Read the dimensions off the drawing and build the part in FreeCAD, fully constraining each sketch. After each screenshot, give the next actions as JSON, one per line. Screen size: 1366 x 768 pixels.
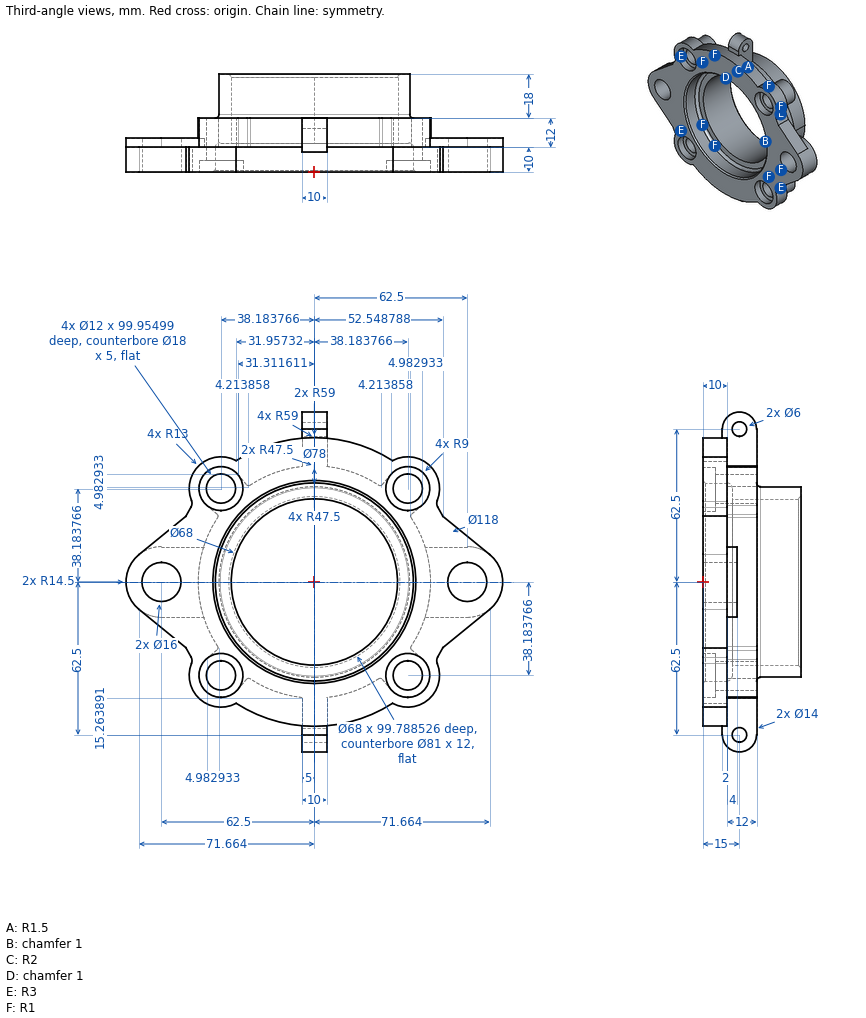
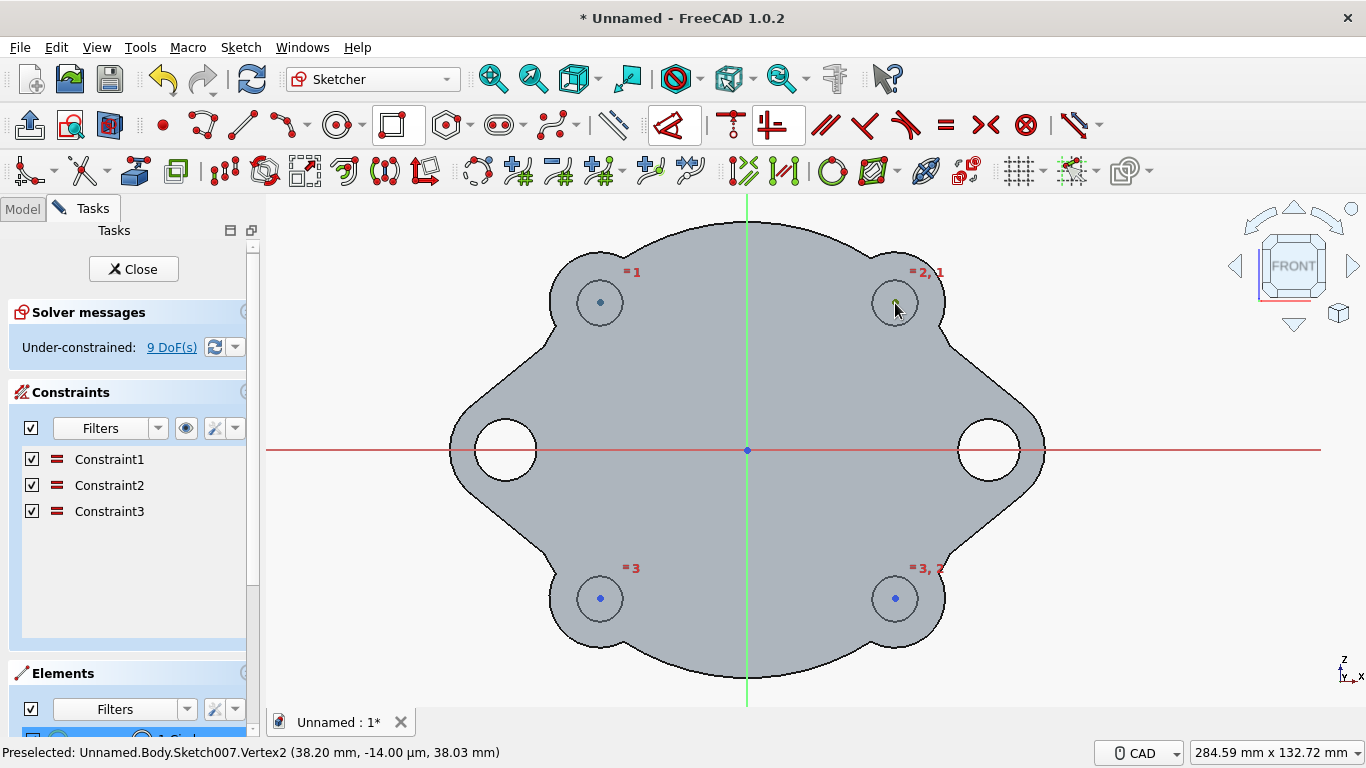
{"action": "key", "text": "h"}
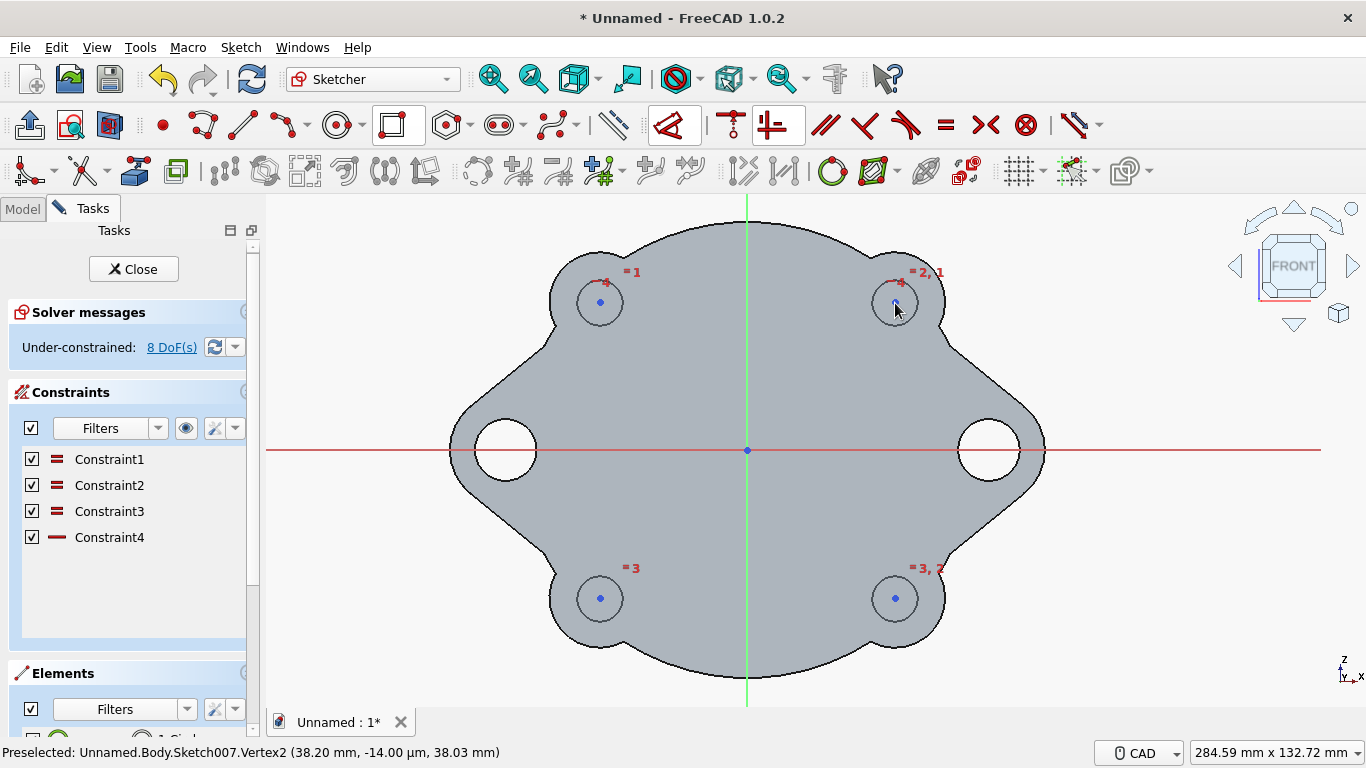
{"action": "left_click", "coordinate": [895, 303]}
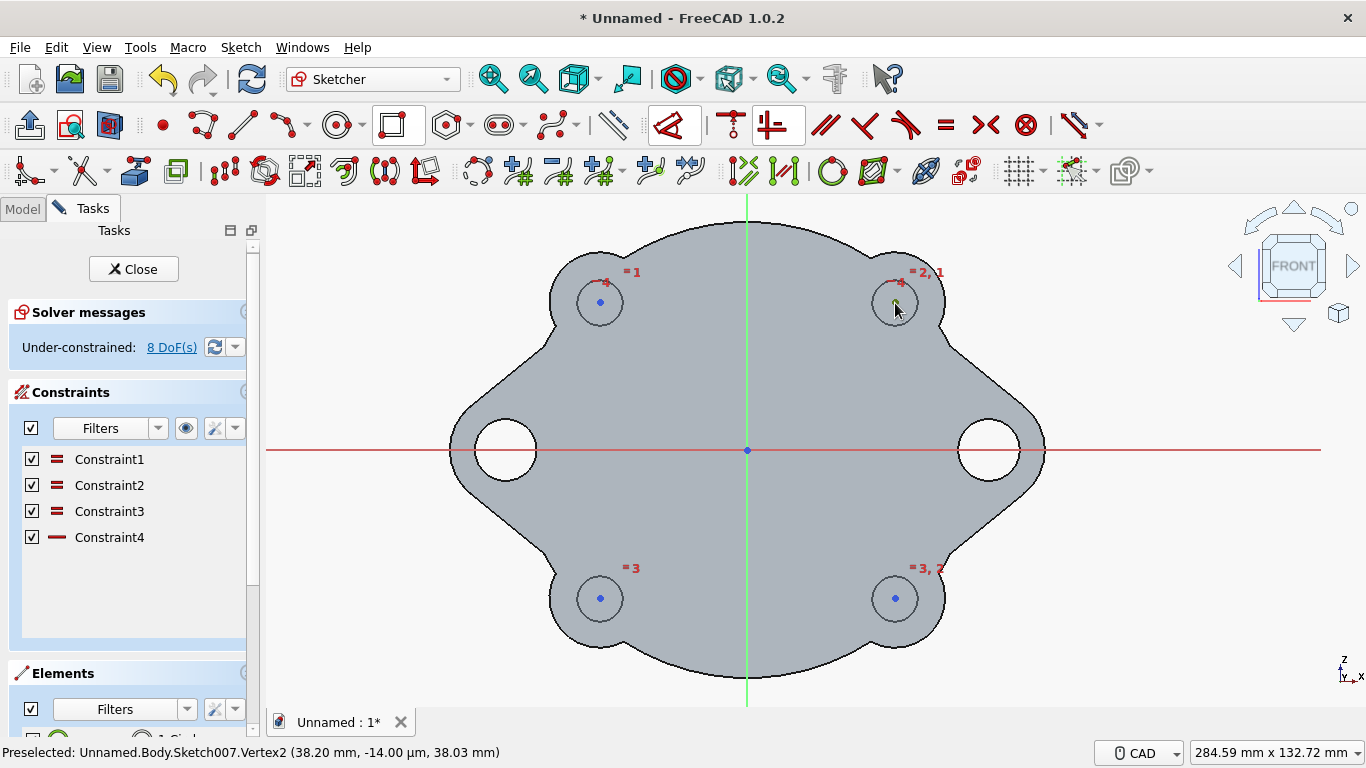
{"action": "left_click", "coordinate": [895, 599]}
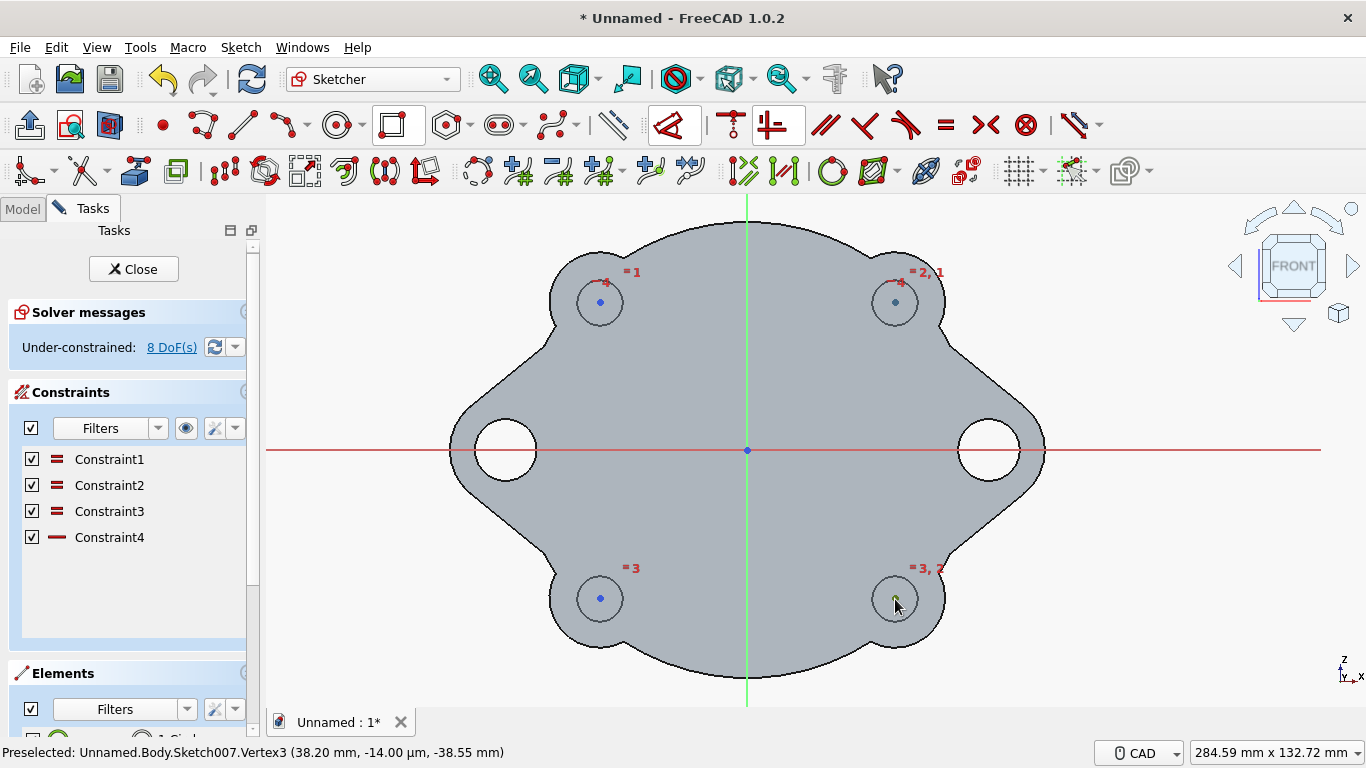
{"action": "key", "text": "v"}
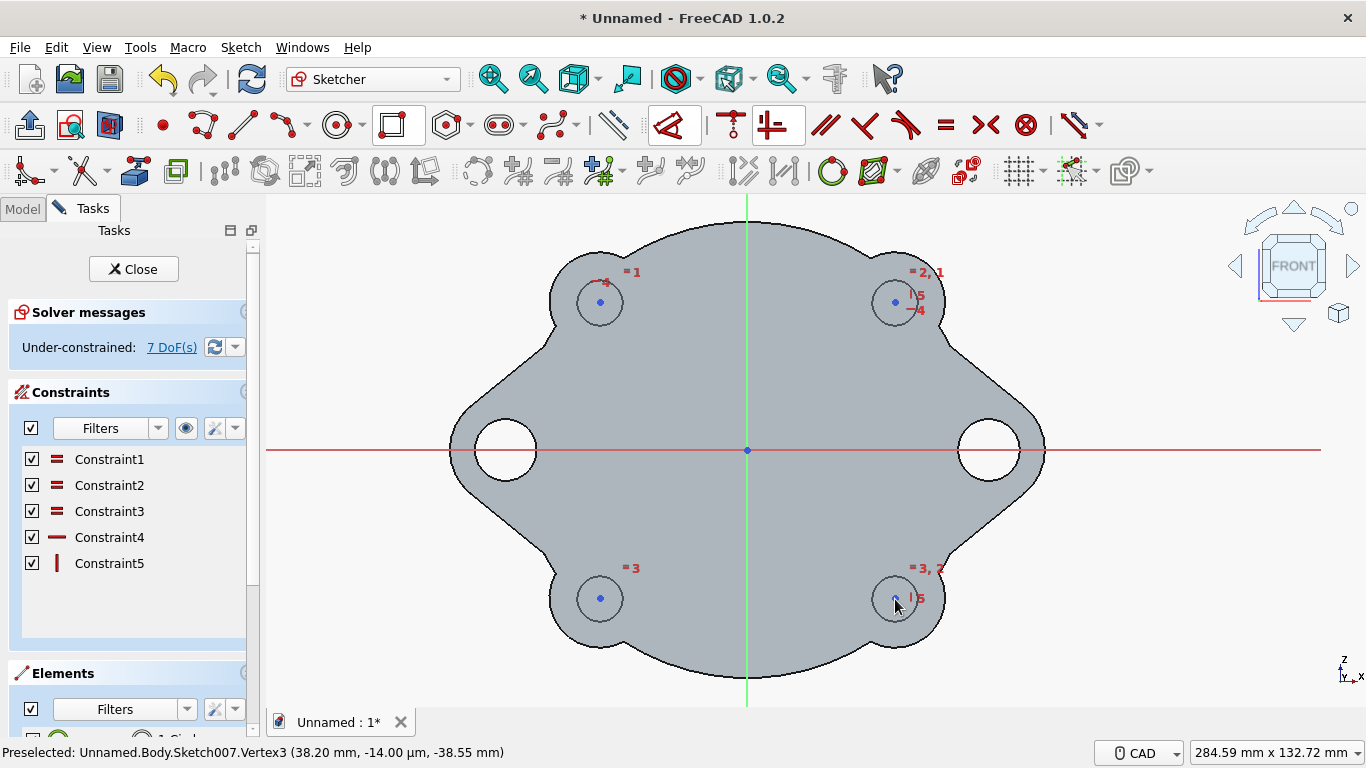
{"action": "left_click", "coordinate": [600, 303]}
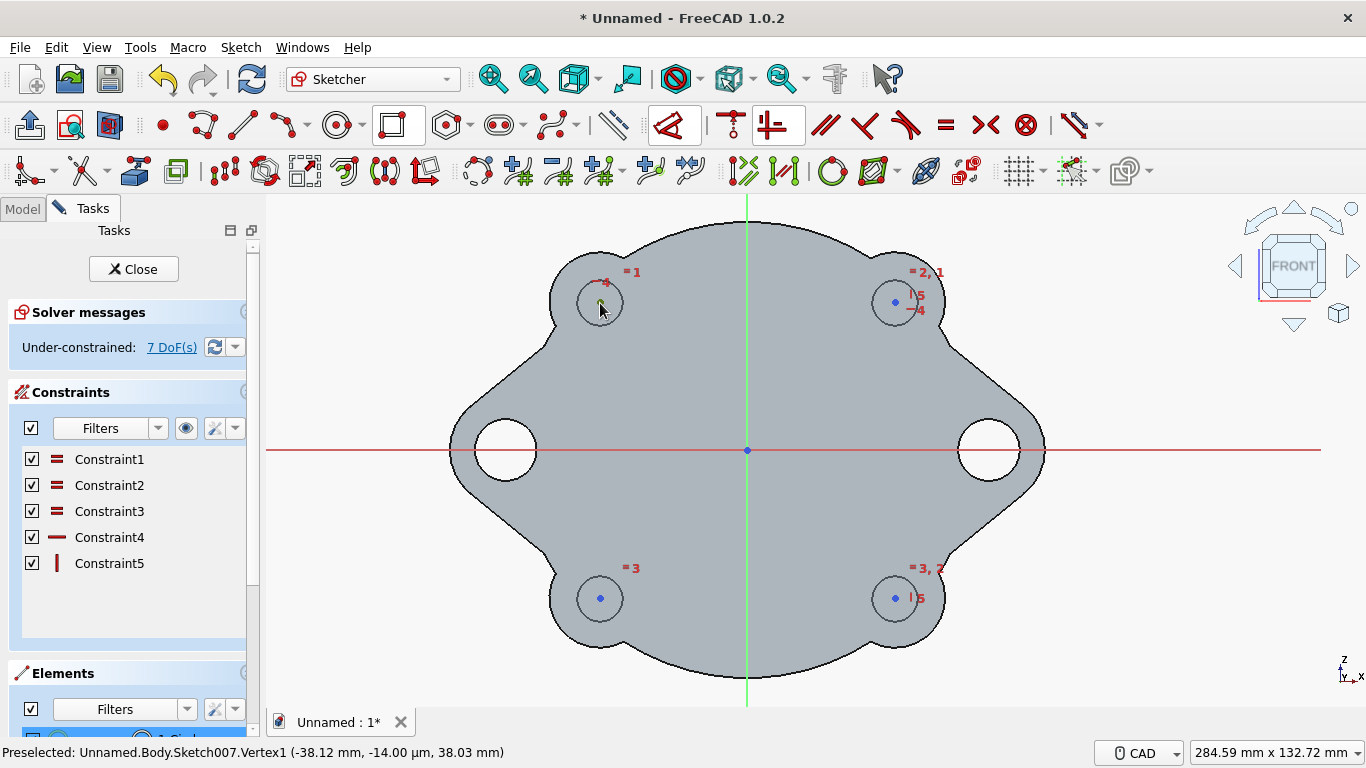
{"action": "left_click", "coordinate": [600, 599]}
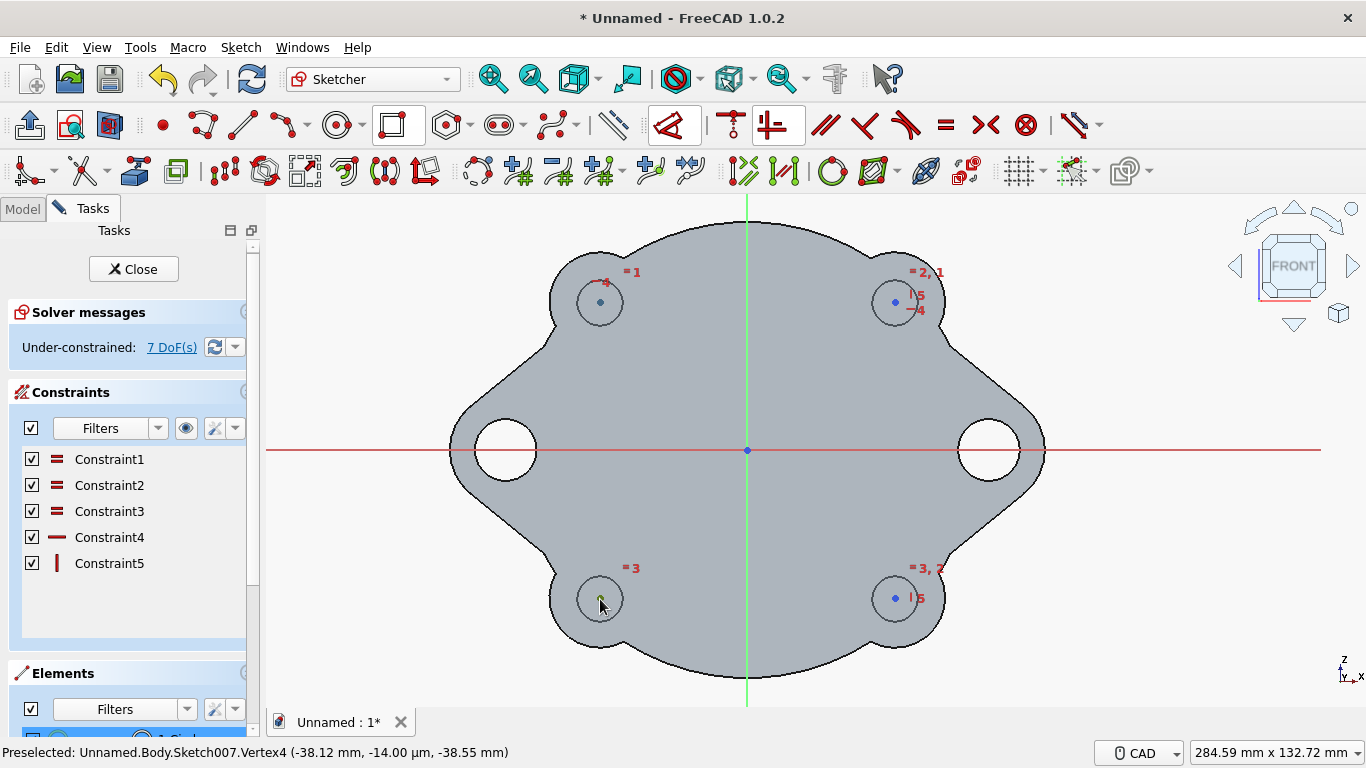
{"action": "key", "text": "v"}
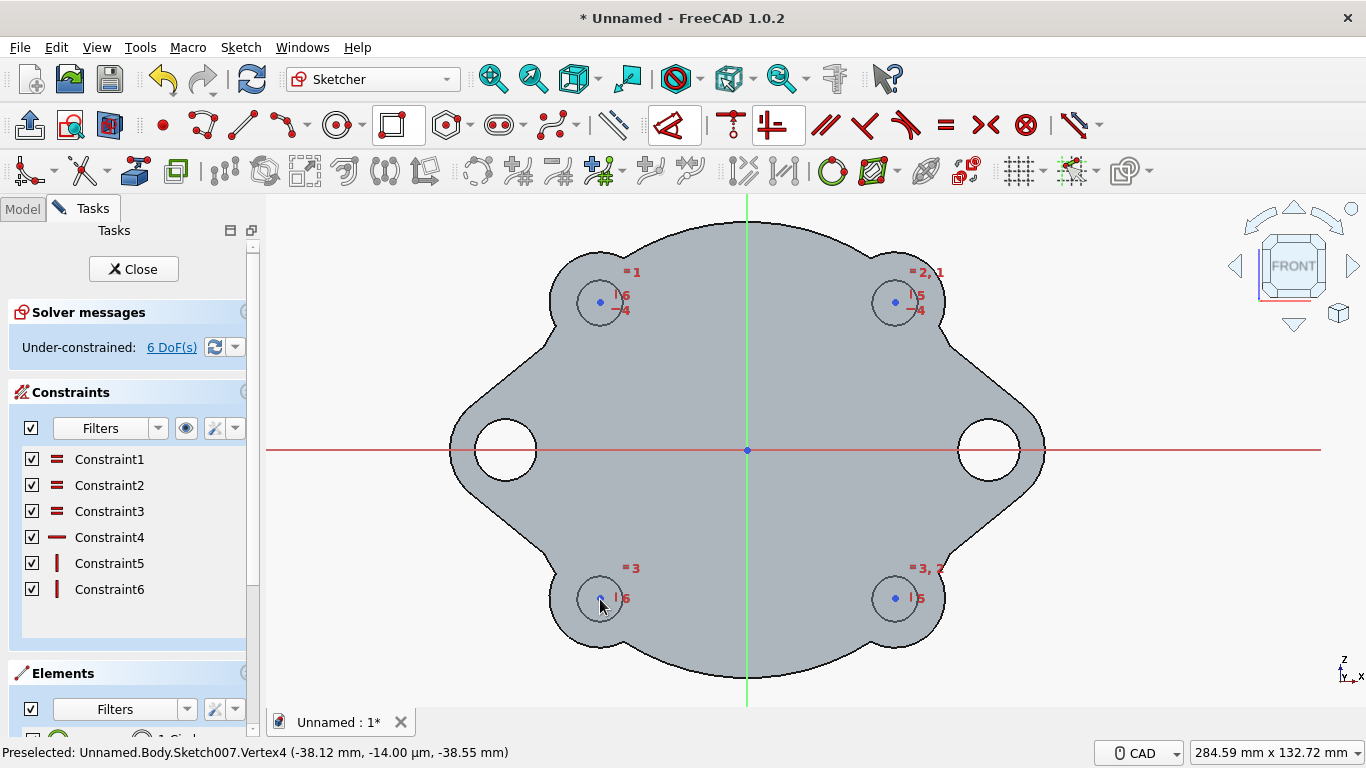
{"action": "left_click", "coordinate": [895, 599]}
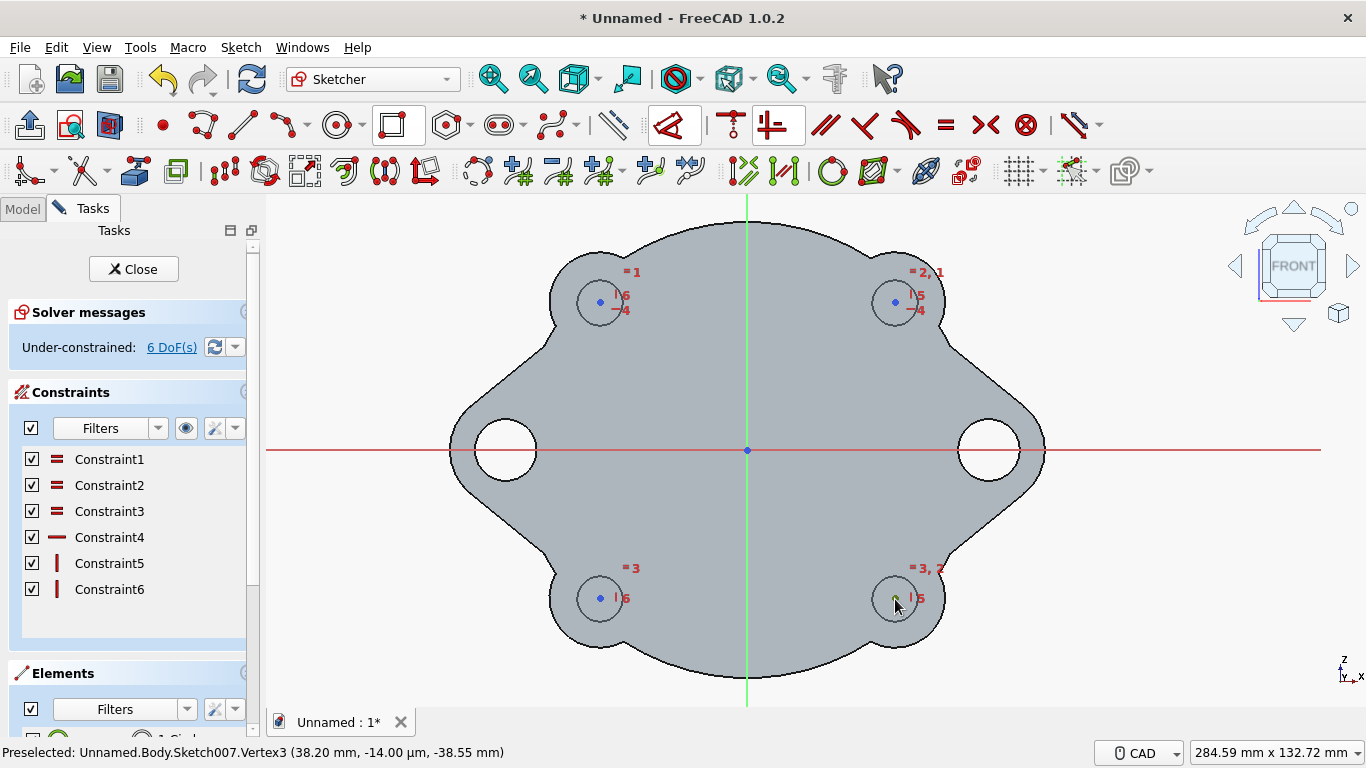
{"action": "left_click", "coordinate": [600, 599]}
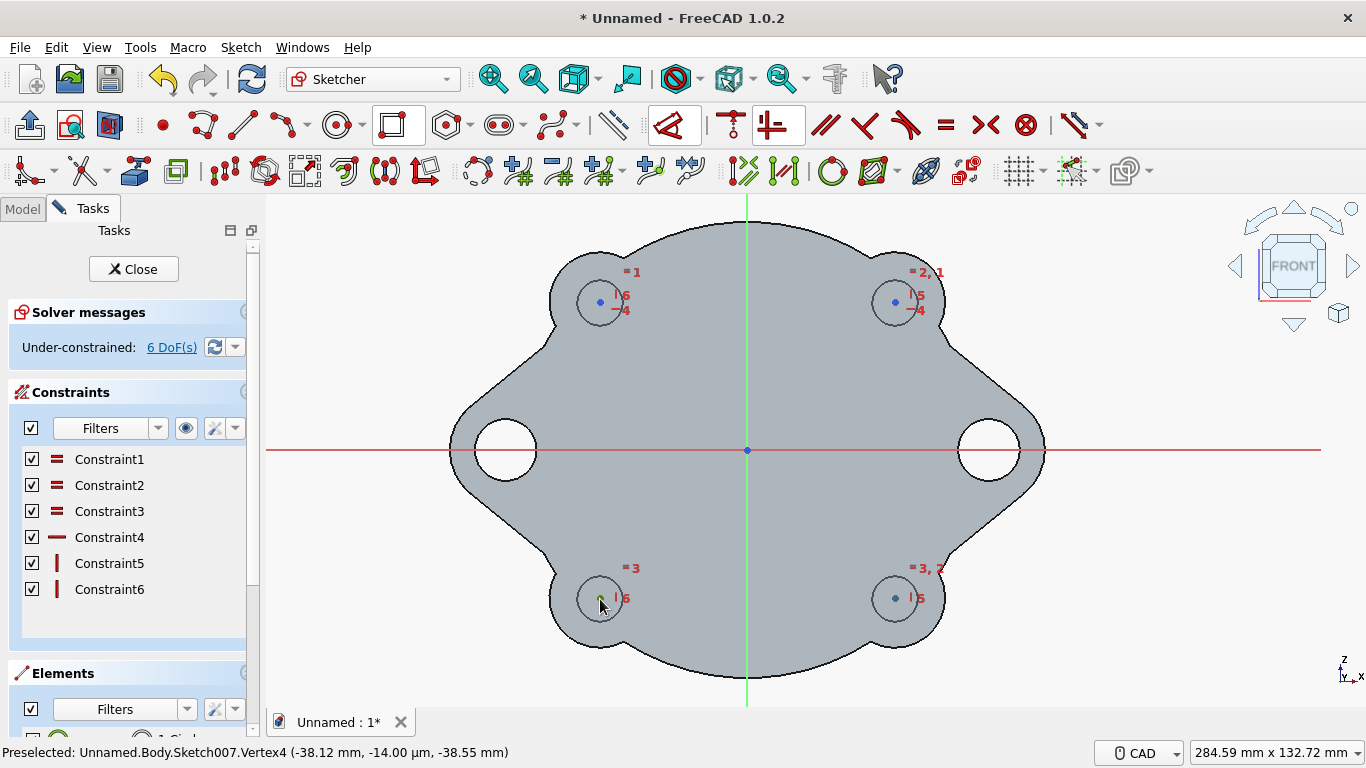
{"action": "left_click", "coordinate": [800, 126]}